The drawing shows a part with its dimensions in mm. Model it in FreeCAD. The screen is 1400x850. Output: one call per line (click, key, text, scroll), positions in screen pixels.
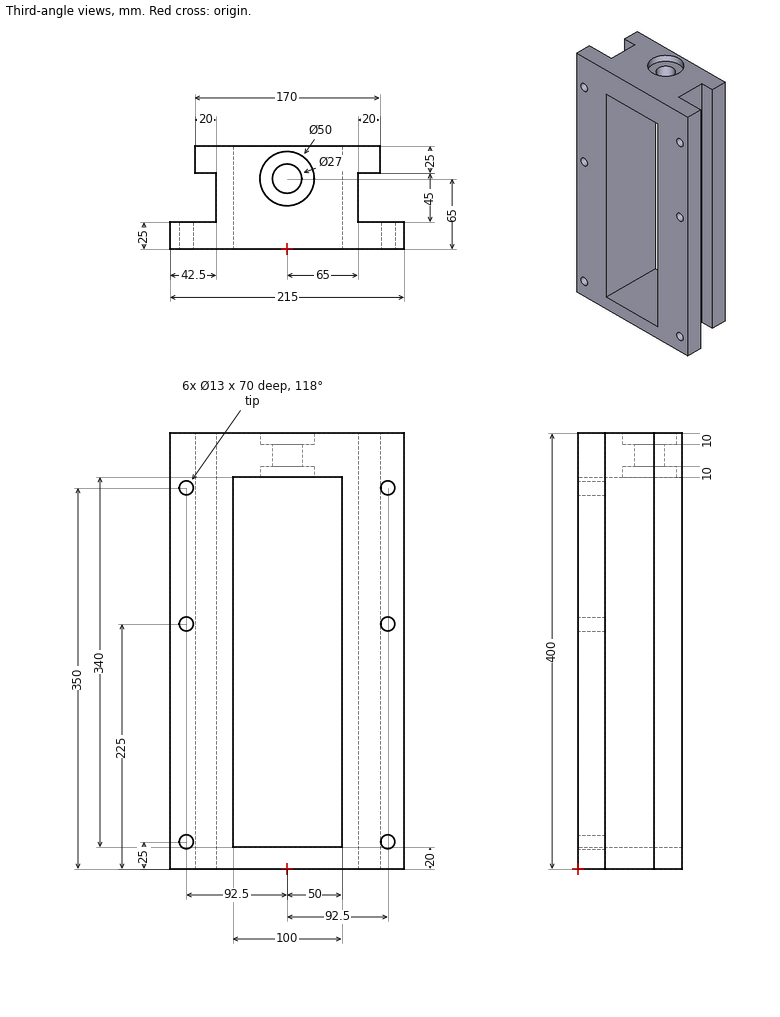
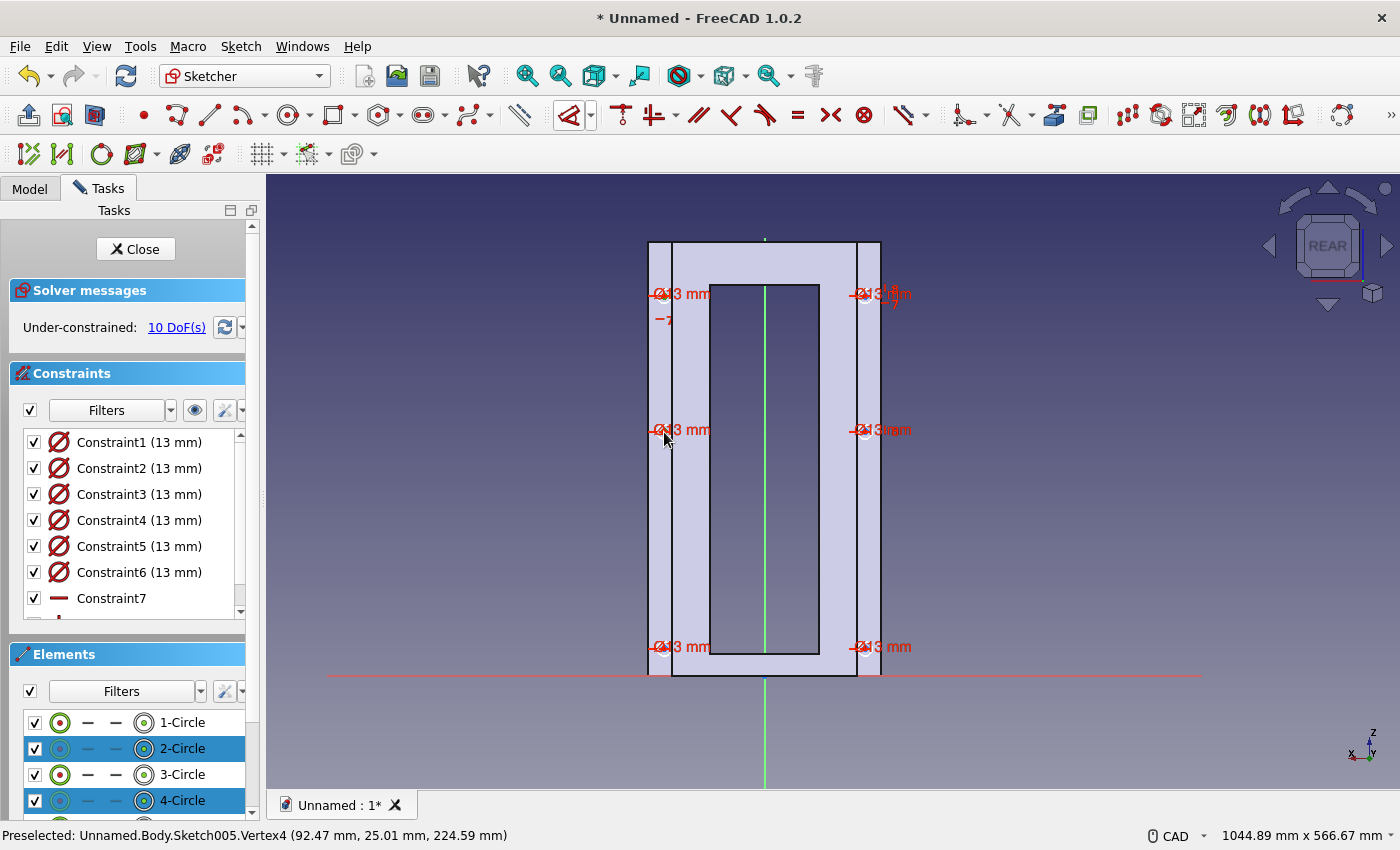
key(v)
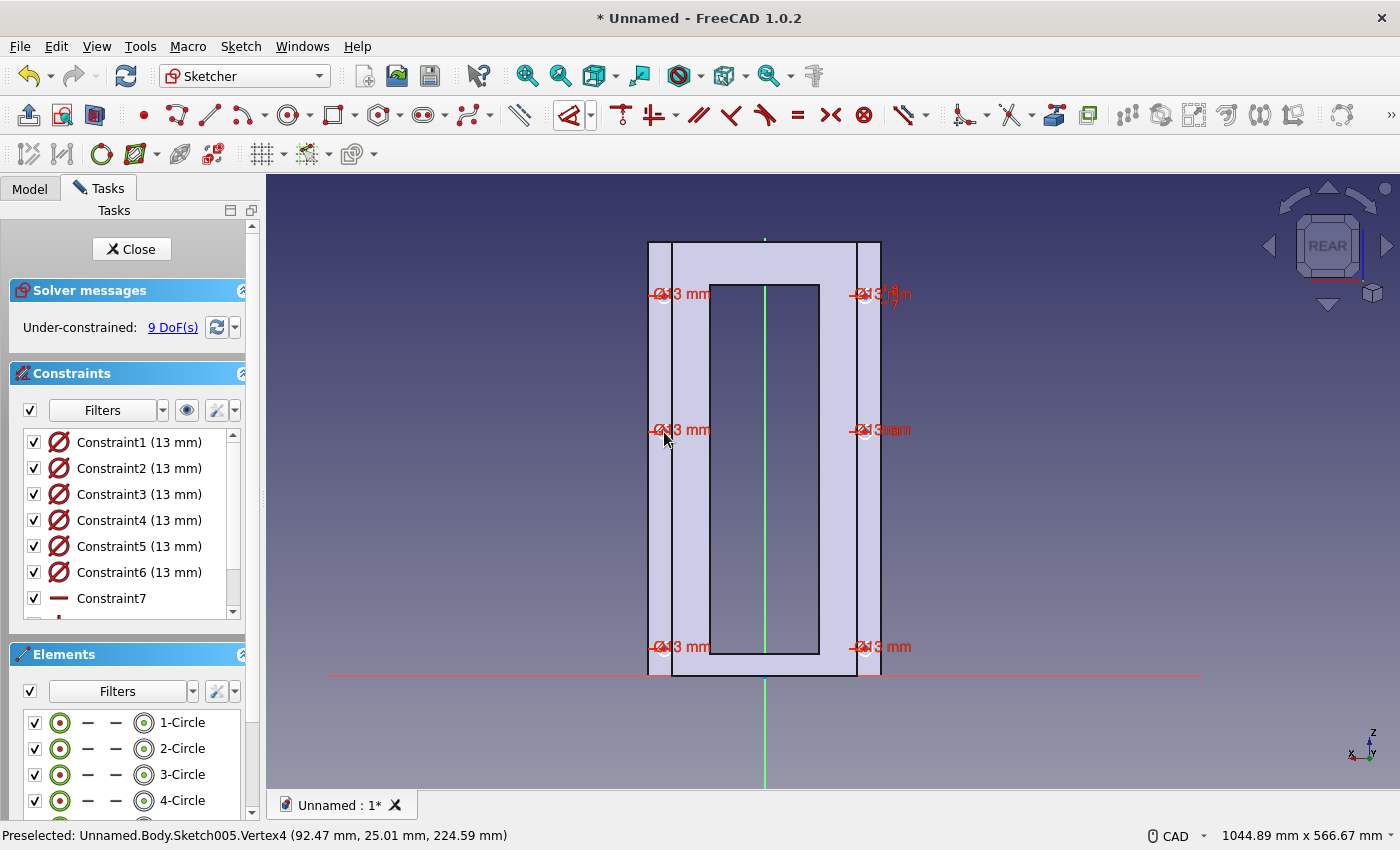
click(865, 432)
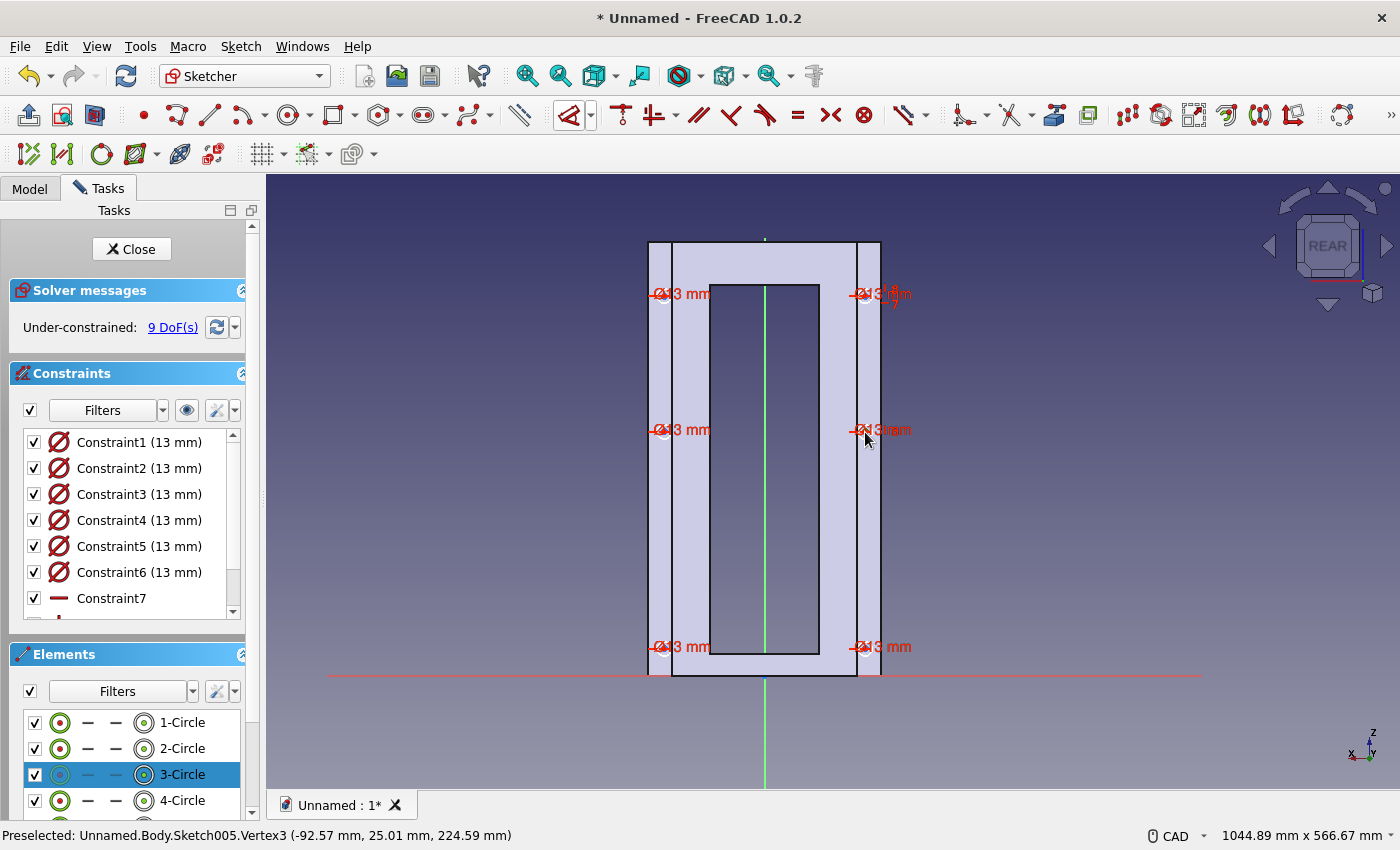
click(664, 432)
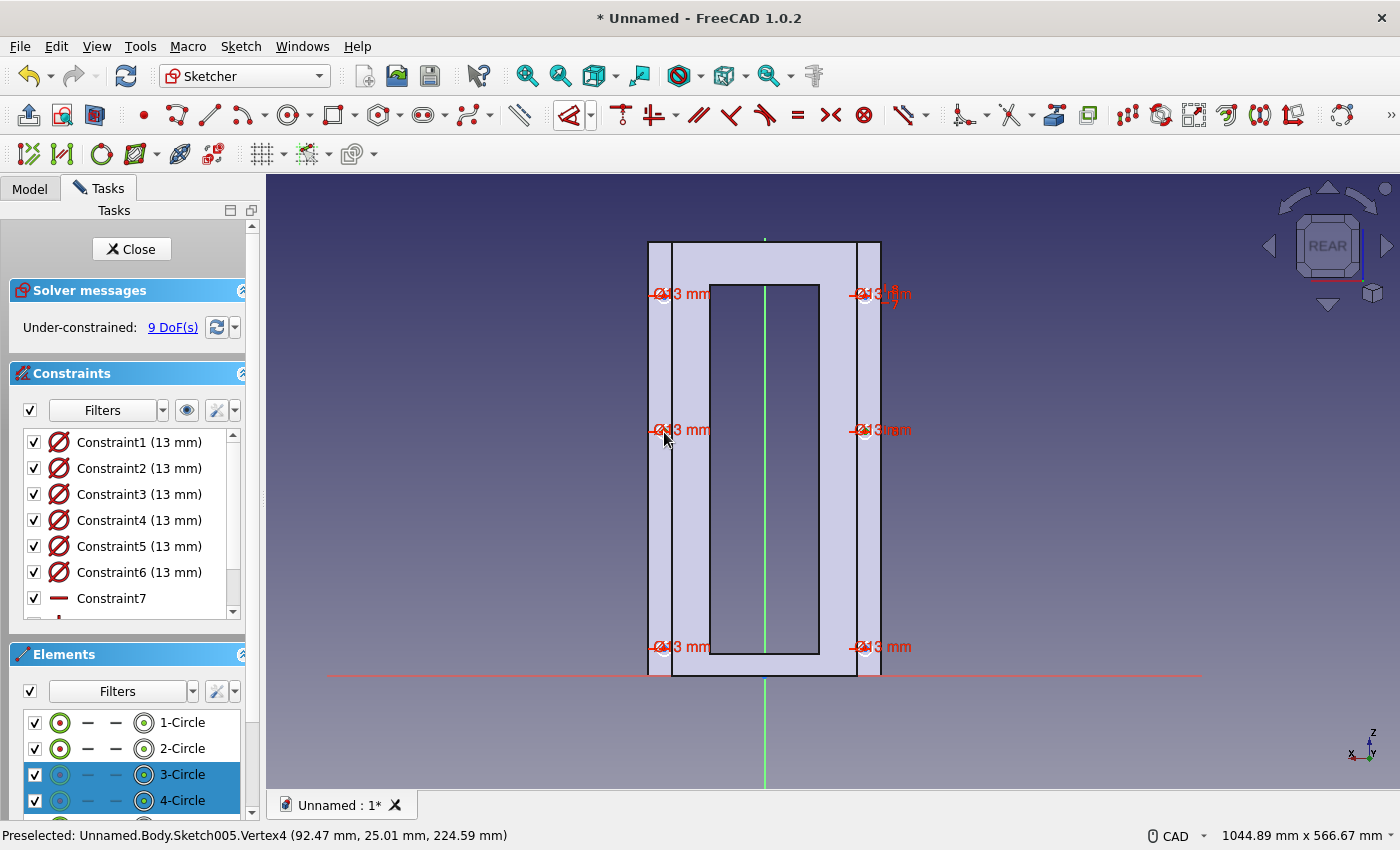
key(h)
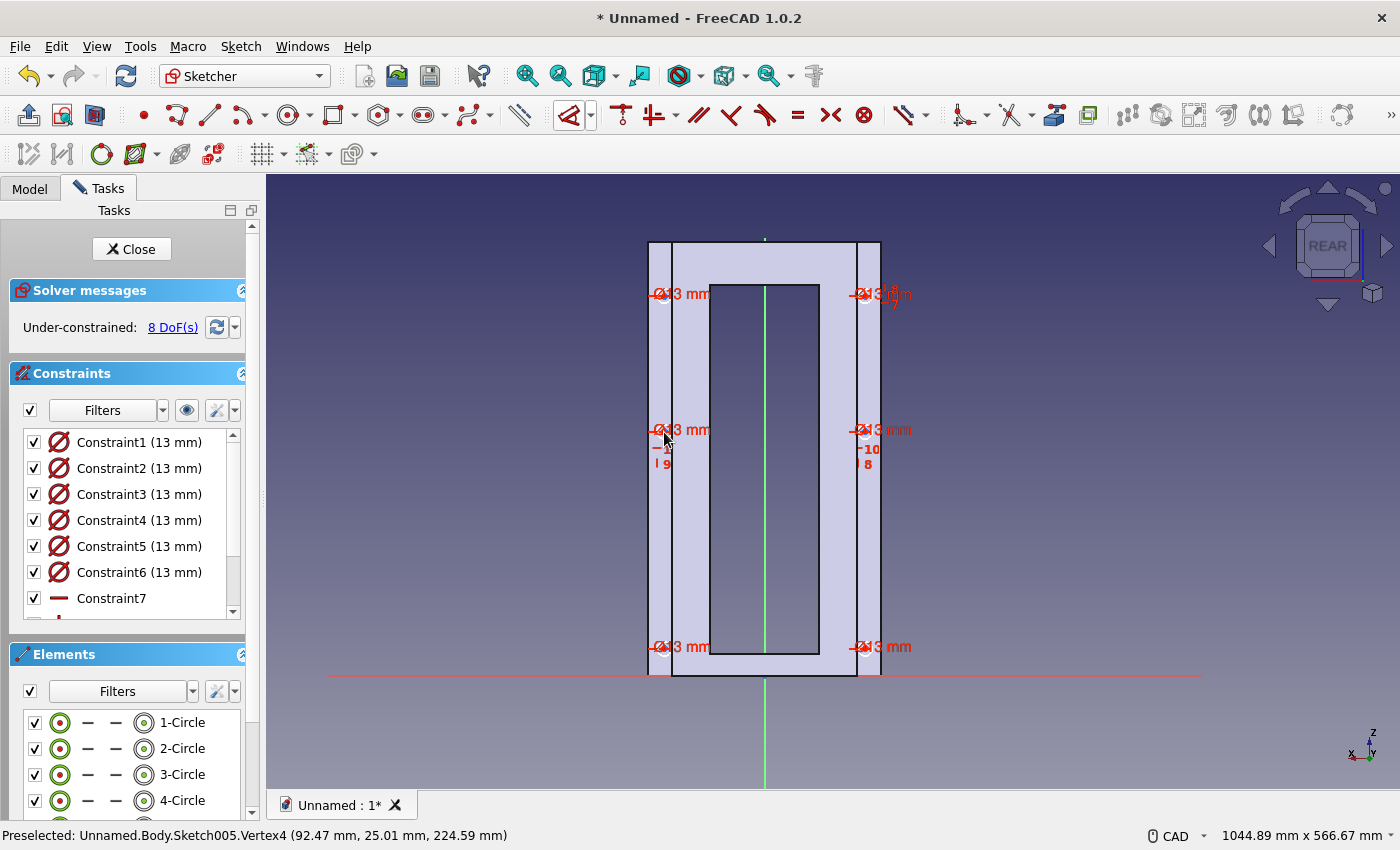
click(865, 432)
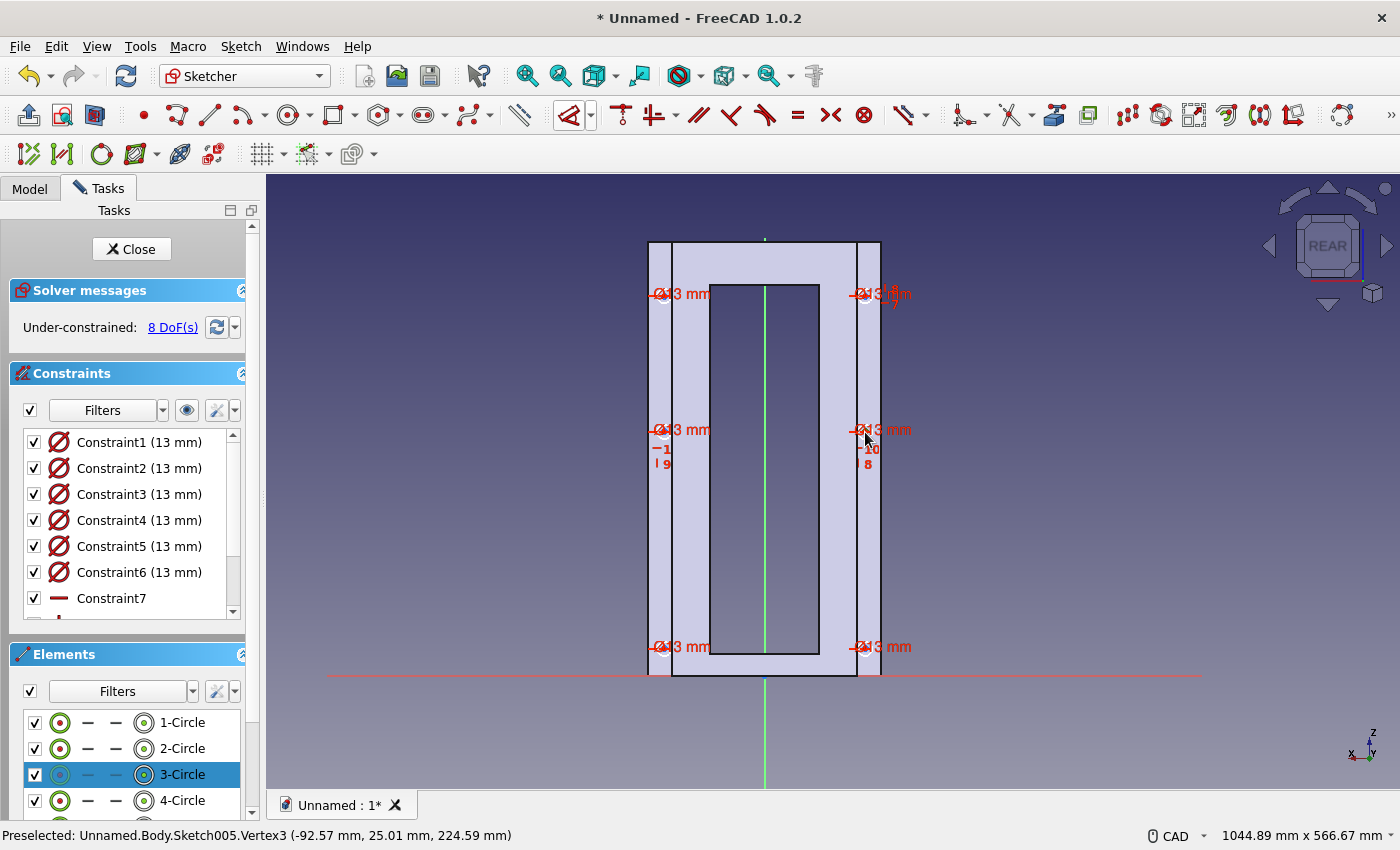
click(865, 649)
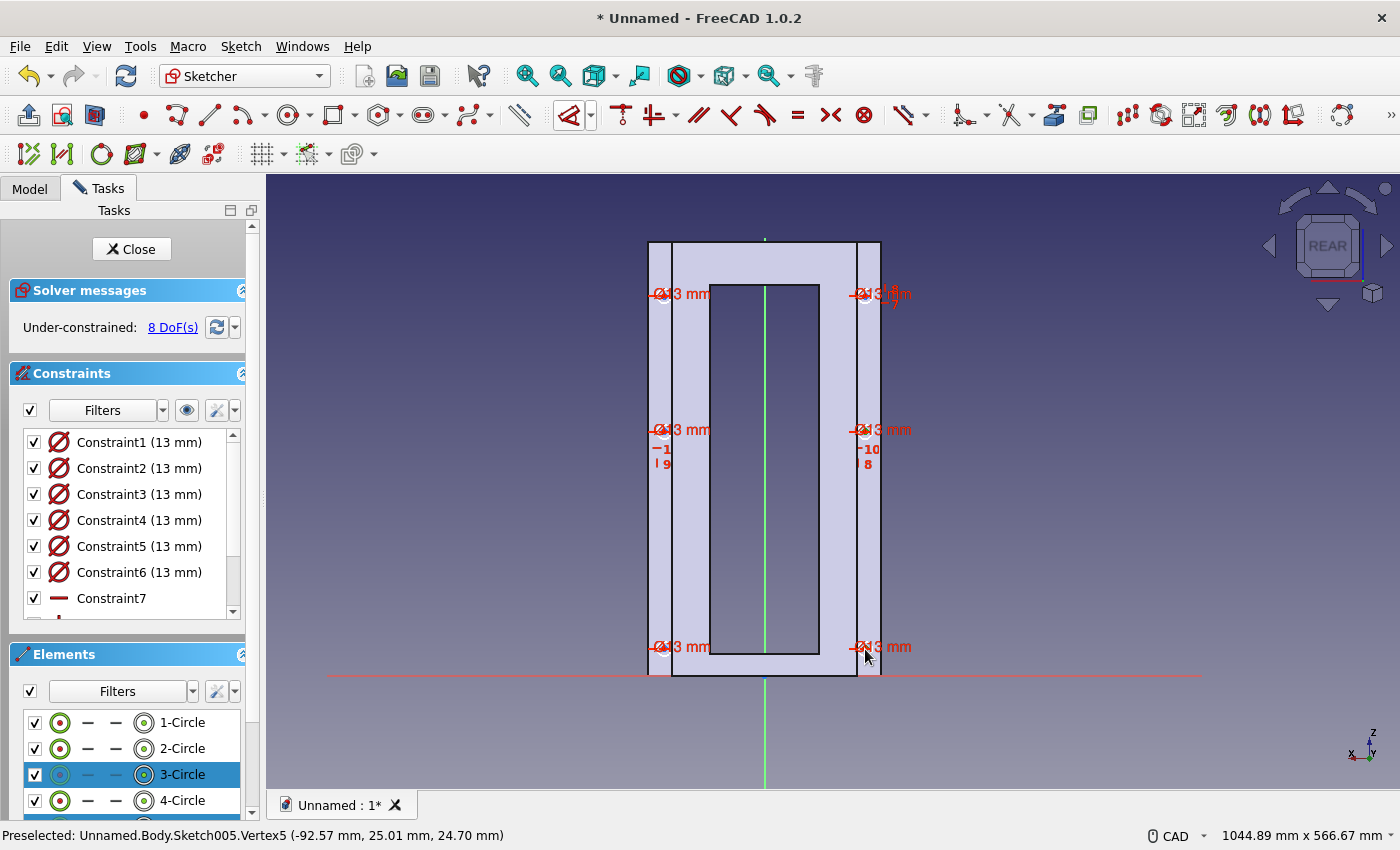
click(676, 116)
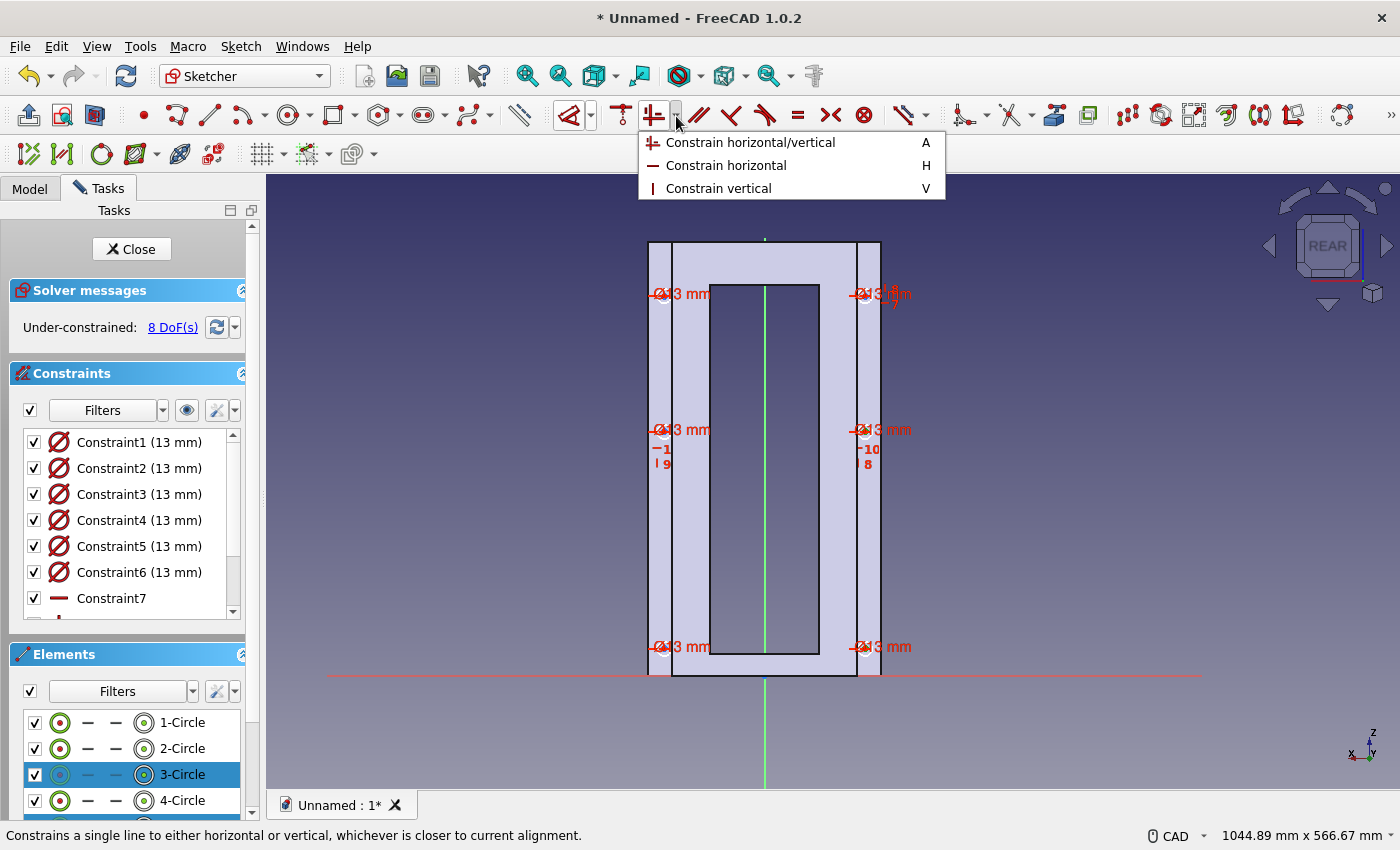
click(792, 188)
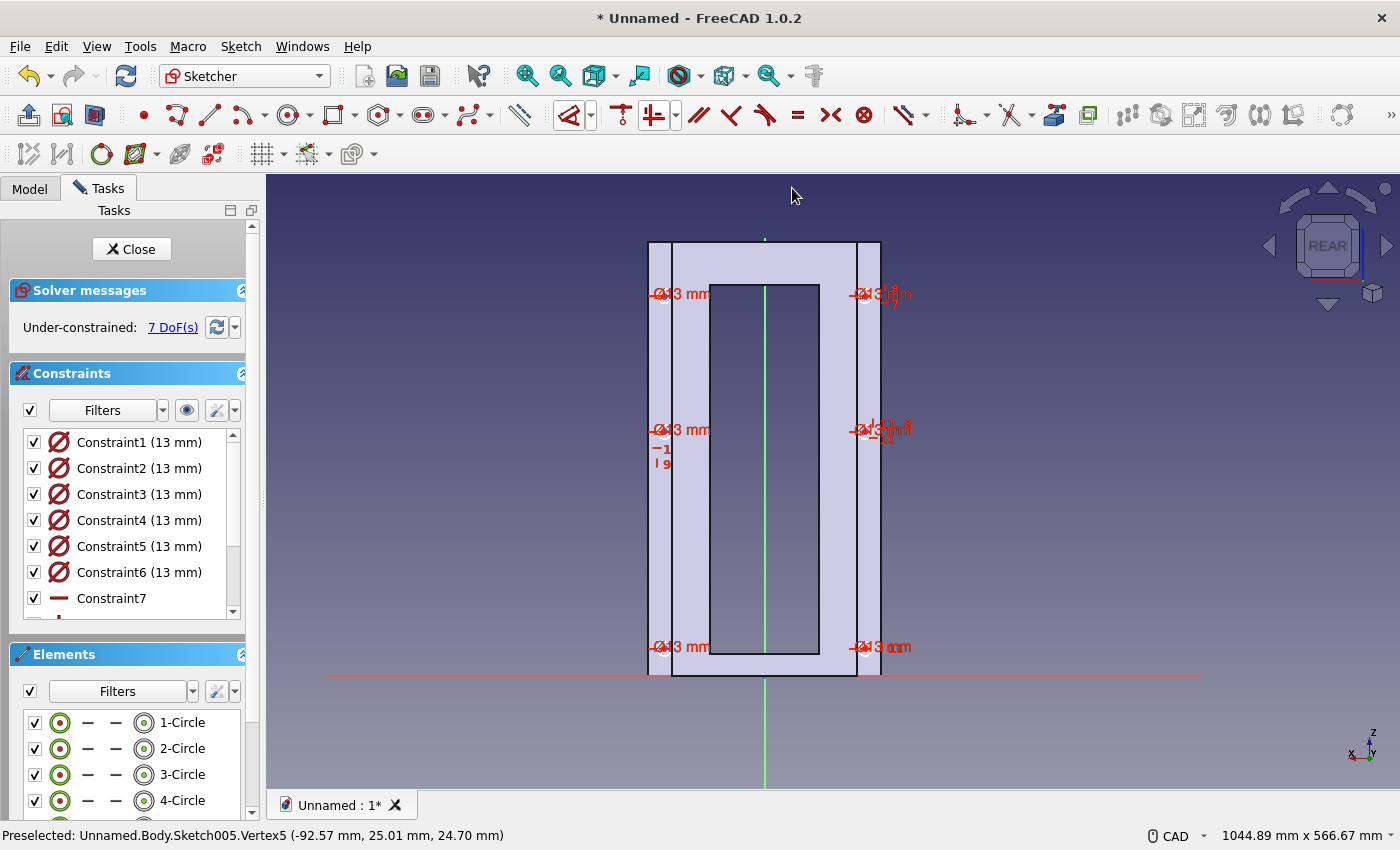
click(664, 432)